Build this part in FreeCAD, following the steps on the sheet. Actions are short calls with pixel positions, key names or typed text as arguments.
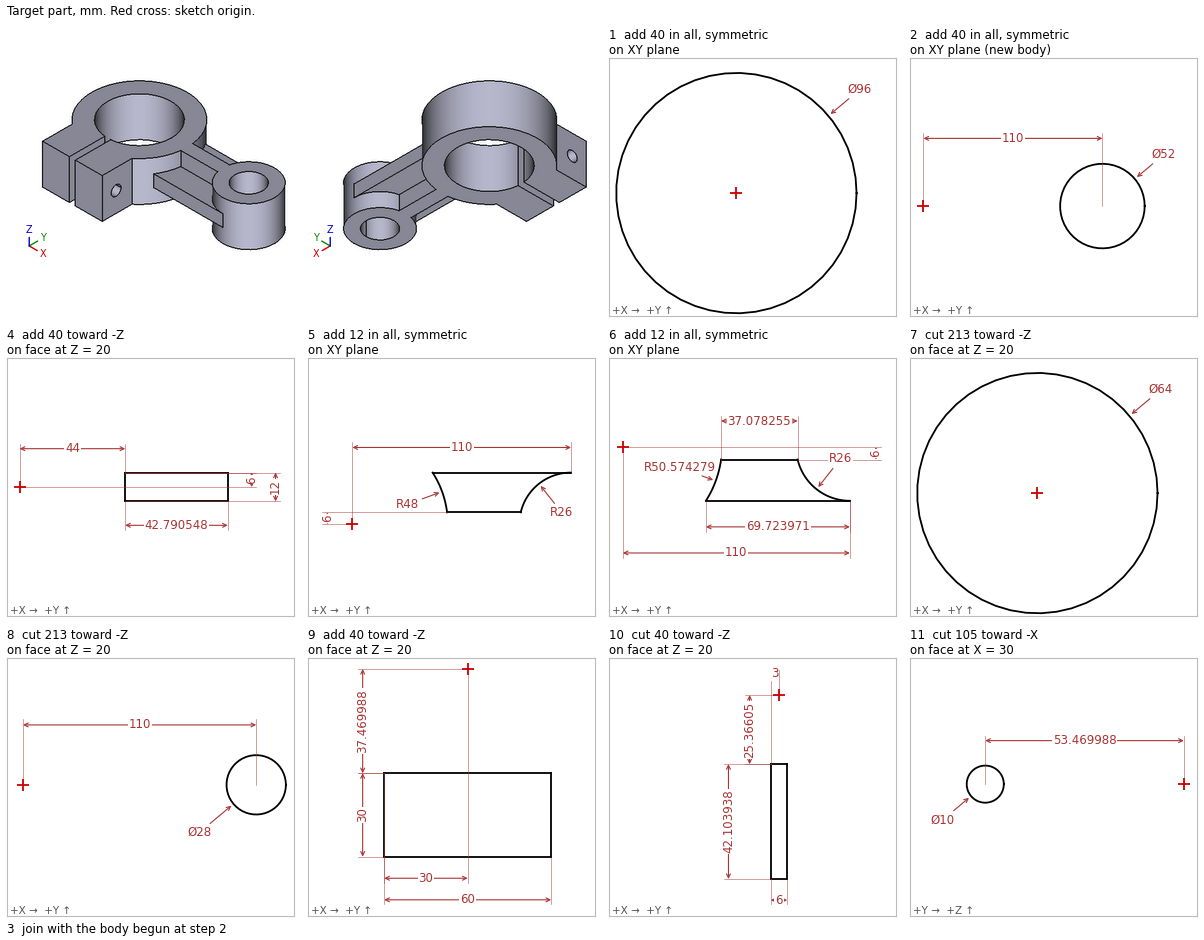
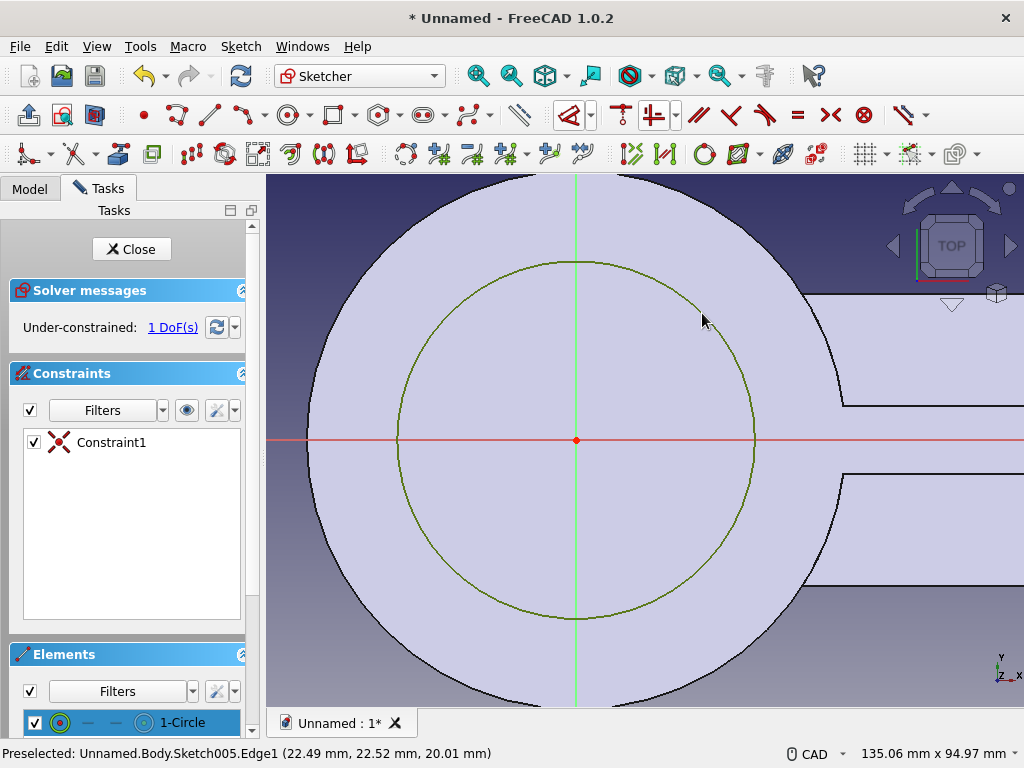
click(590, 116)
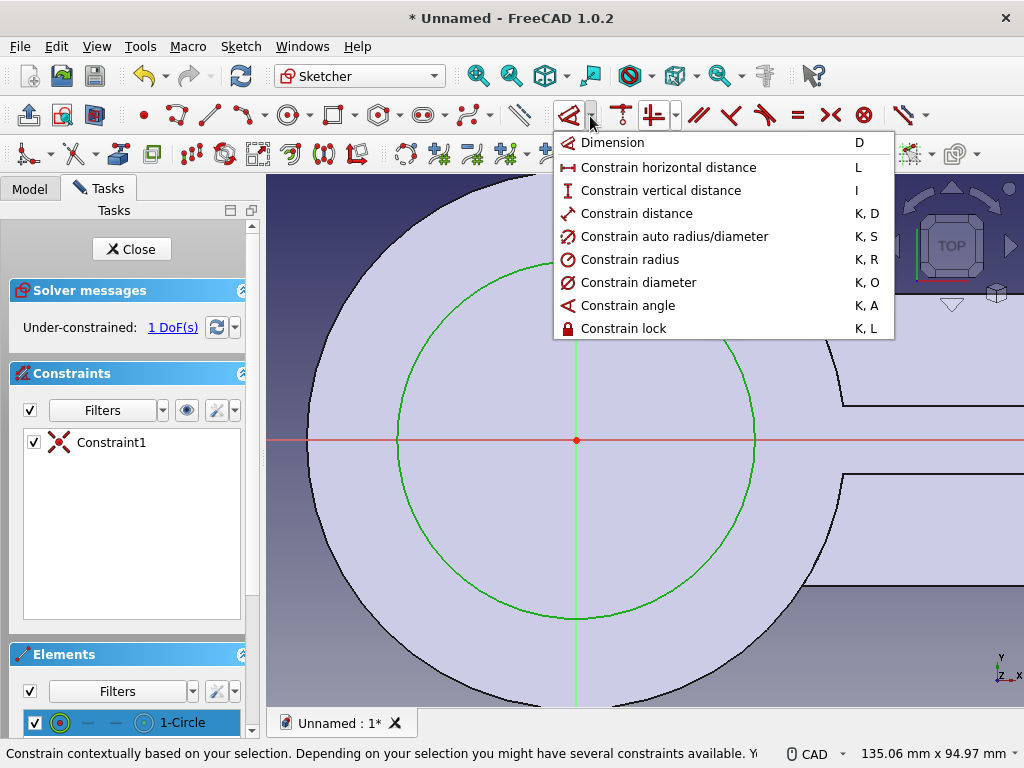
click(724, 282)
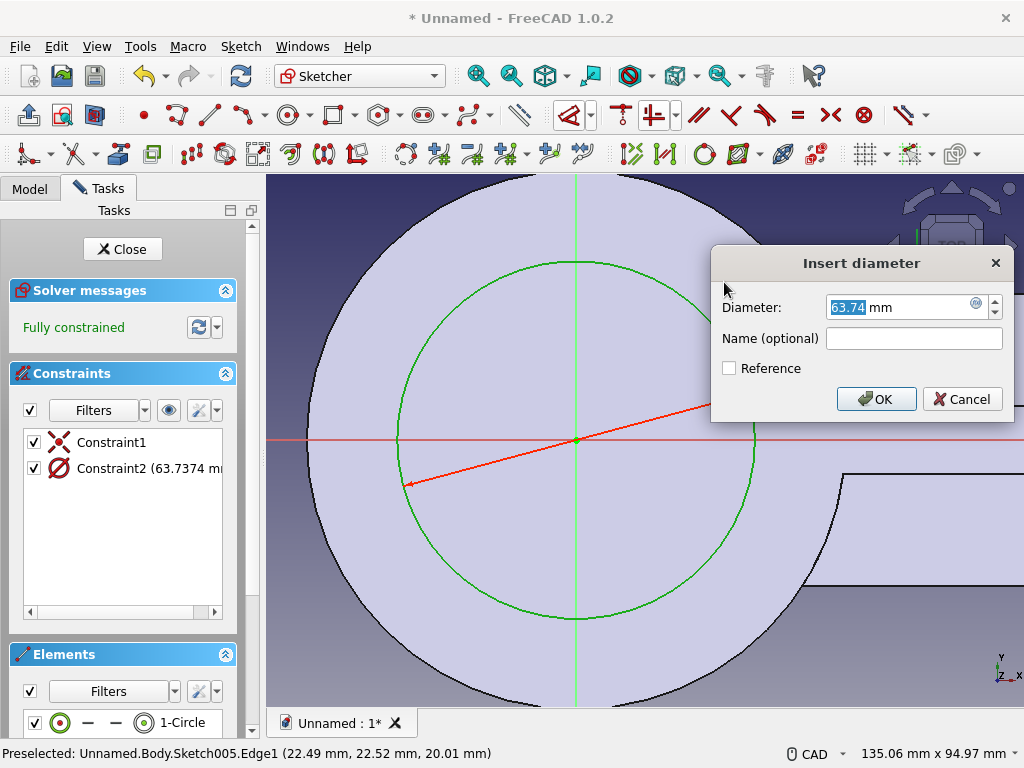
text(64)
key(Return)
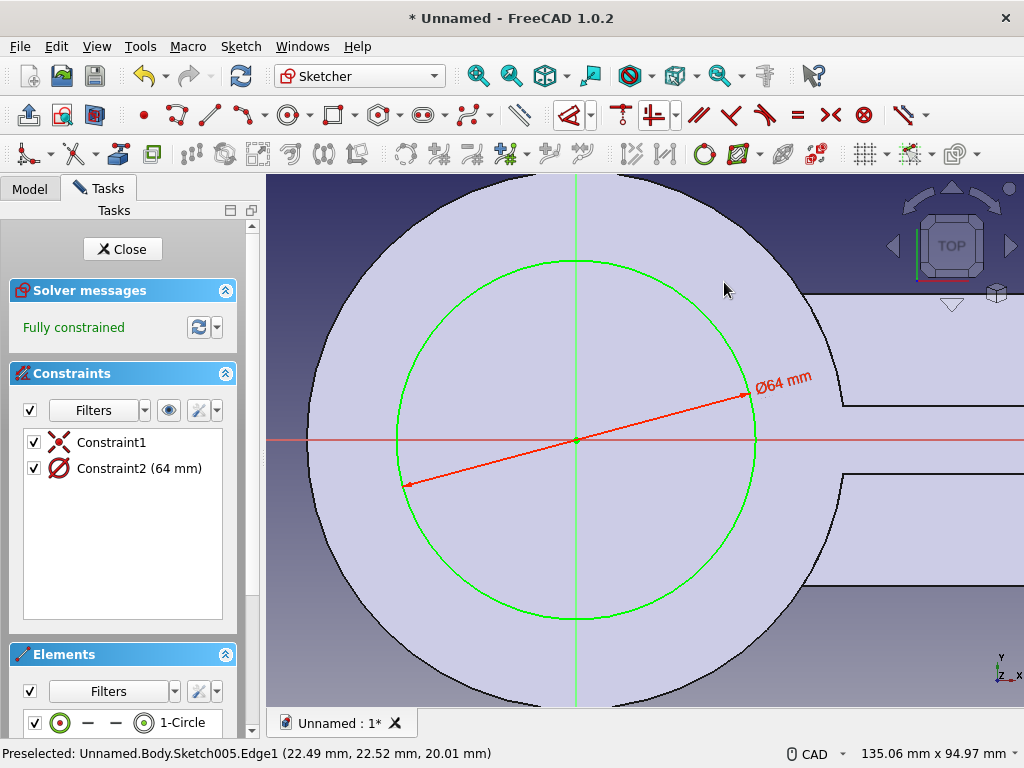
click(123, 249)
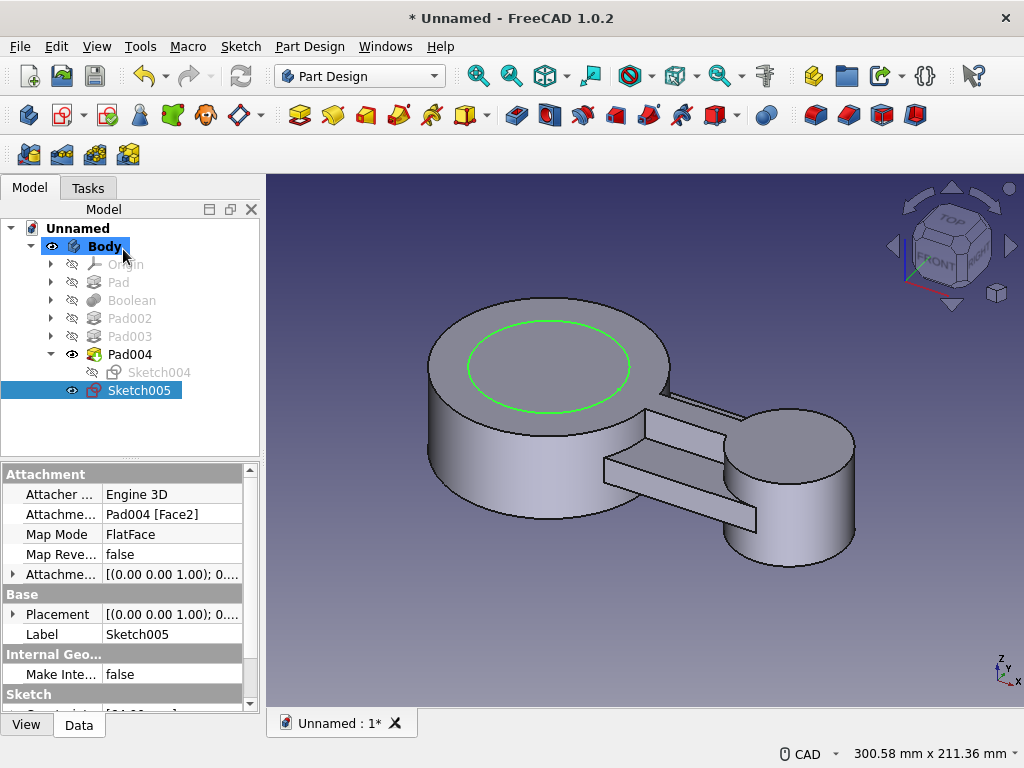
click(517, 116)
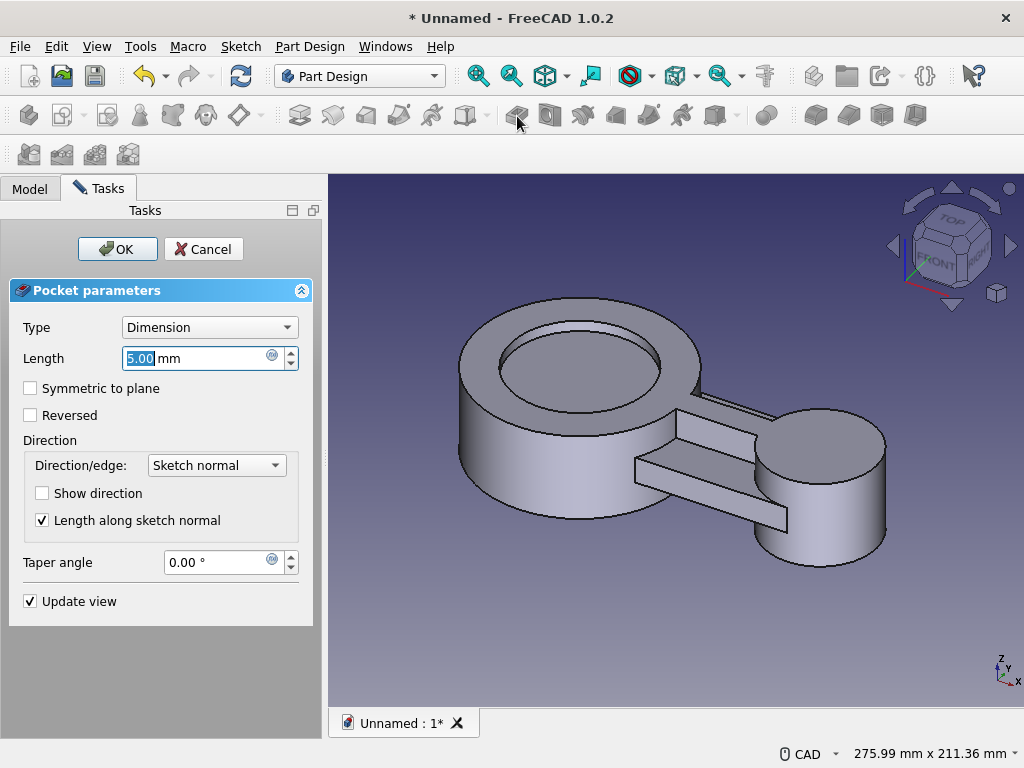
text(213)
key(Tab)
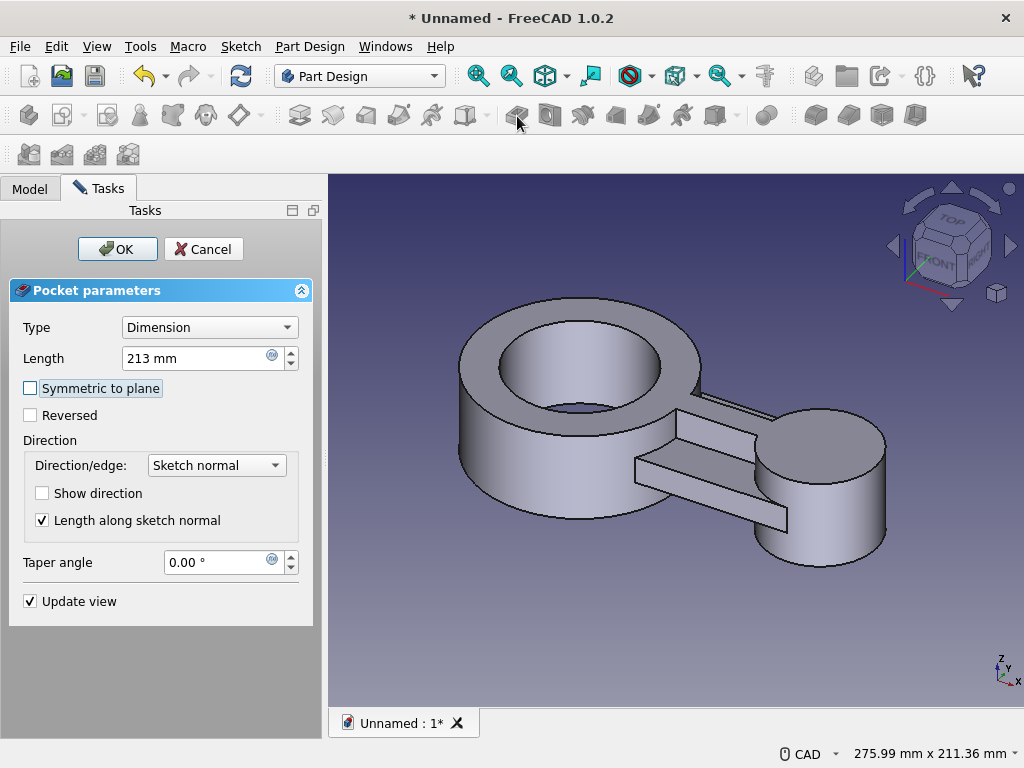
click(118, 249)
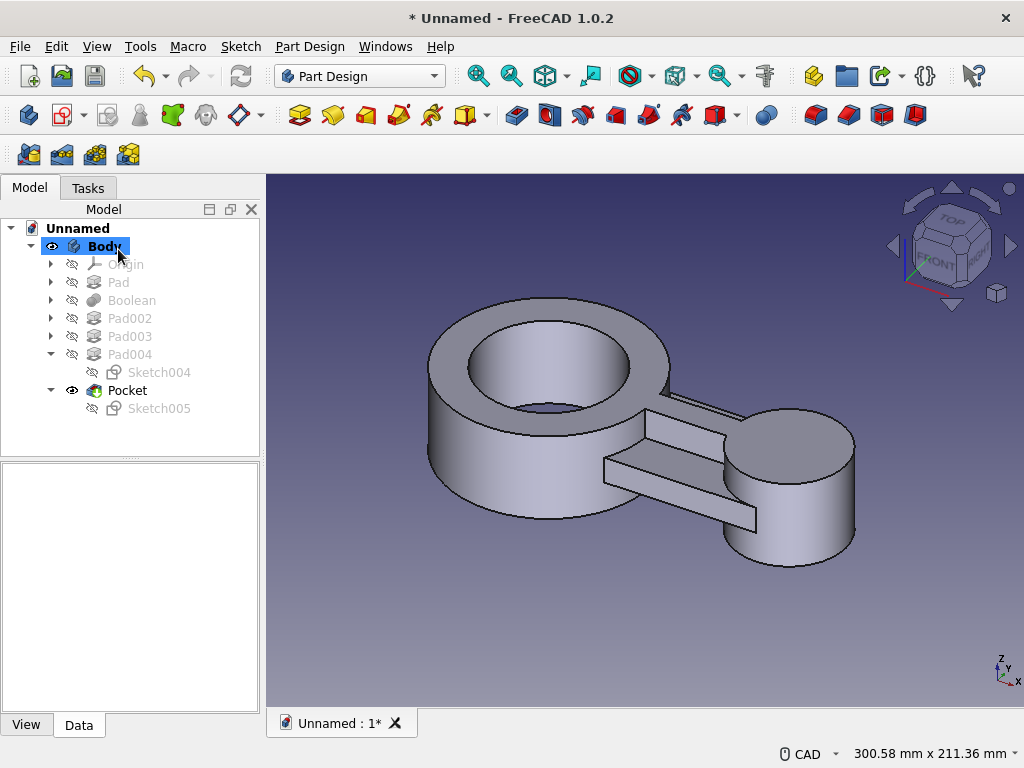
click(760, 436)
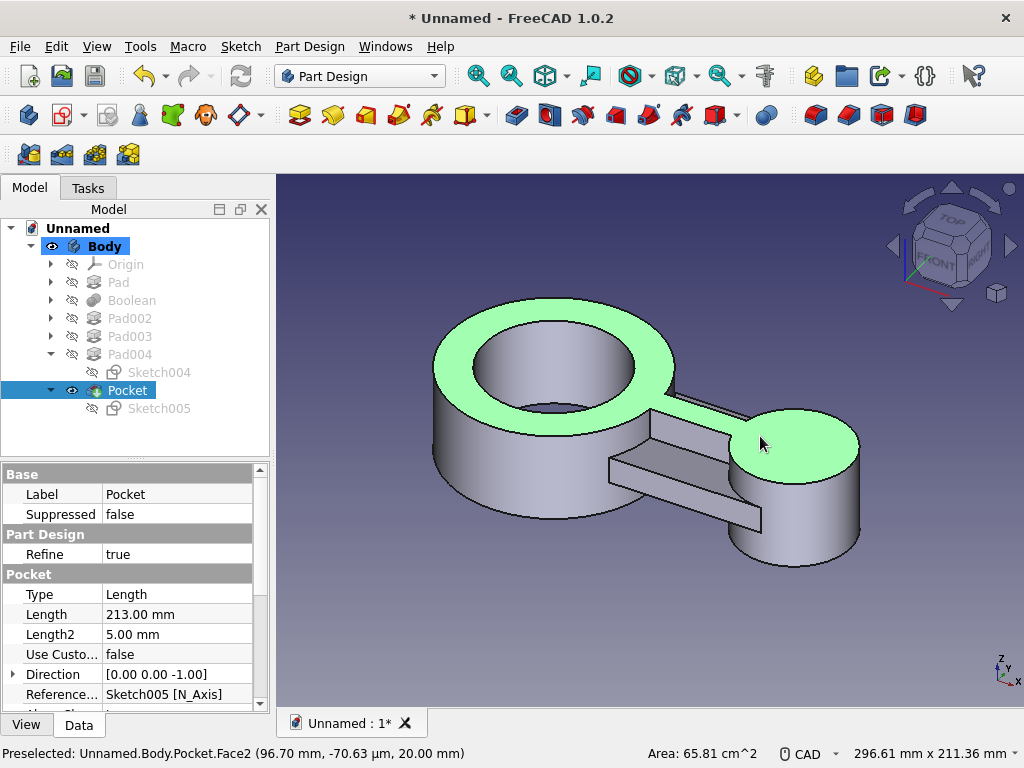
click(62, 116)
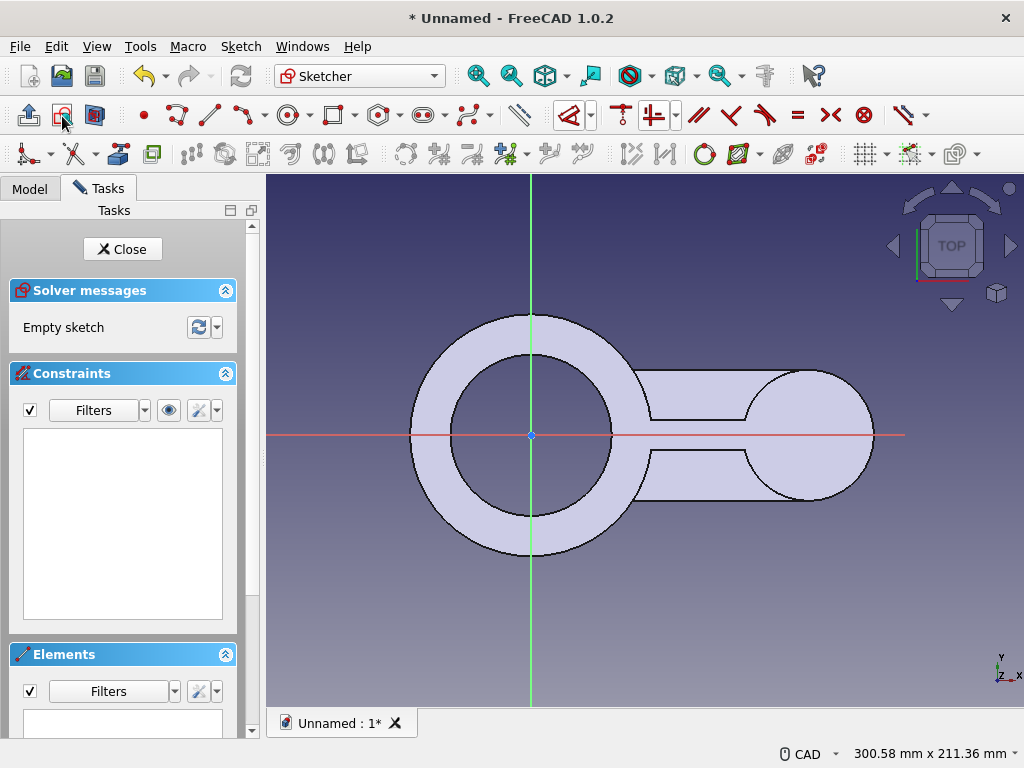
scroll(859, 434, up, 8)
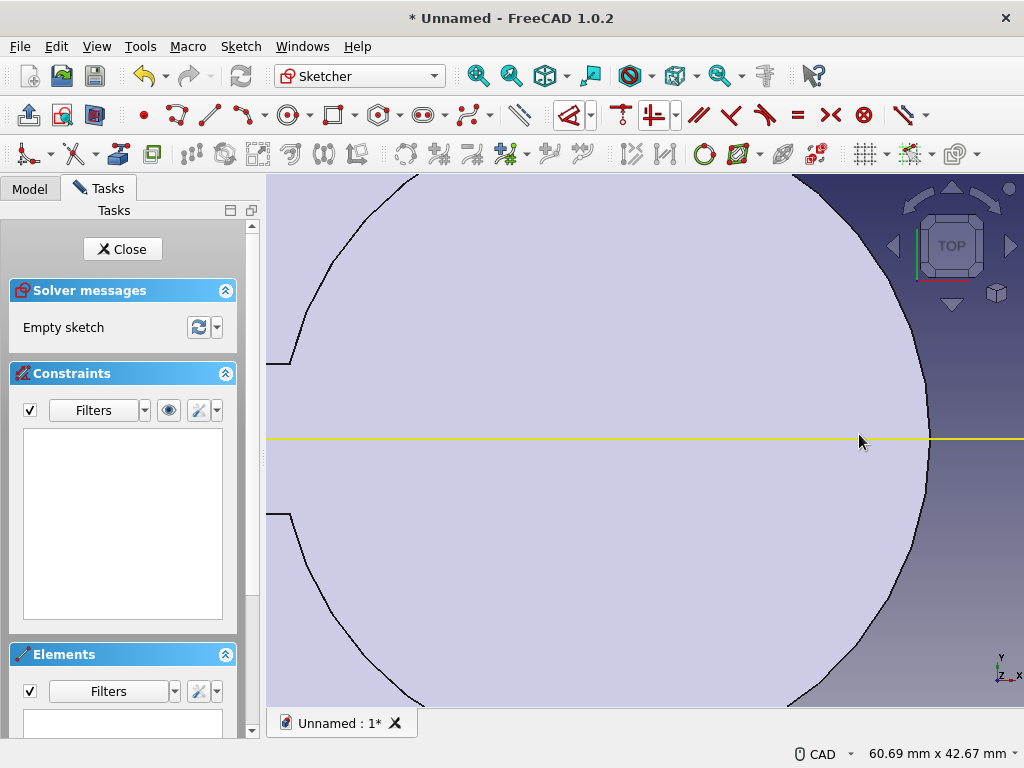
click(288, 116)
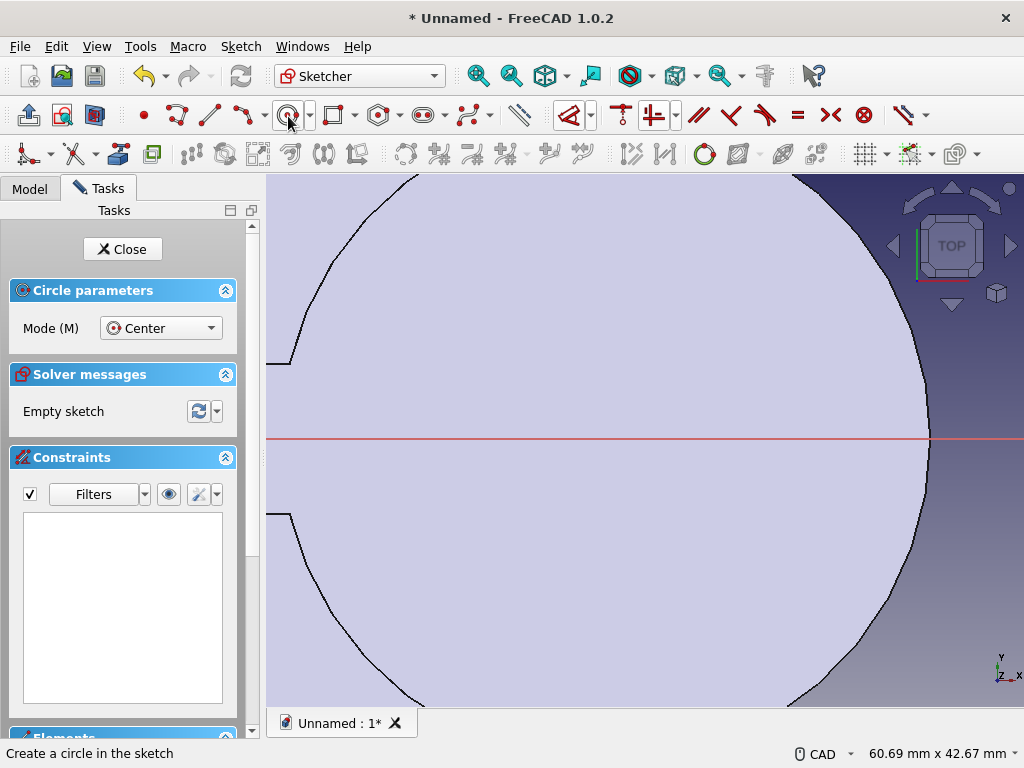
click(606, 439)
click(729, 315)
key(Escape)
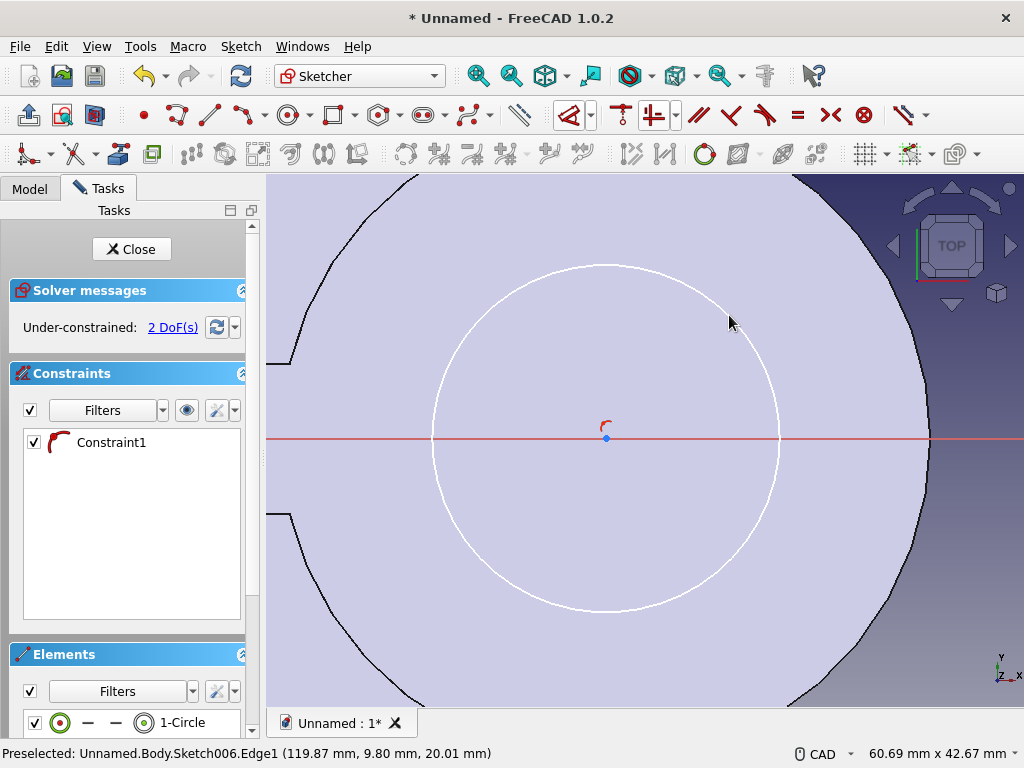
click(728, 315)